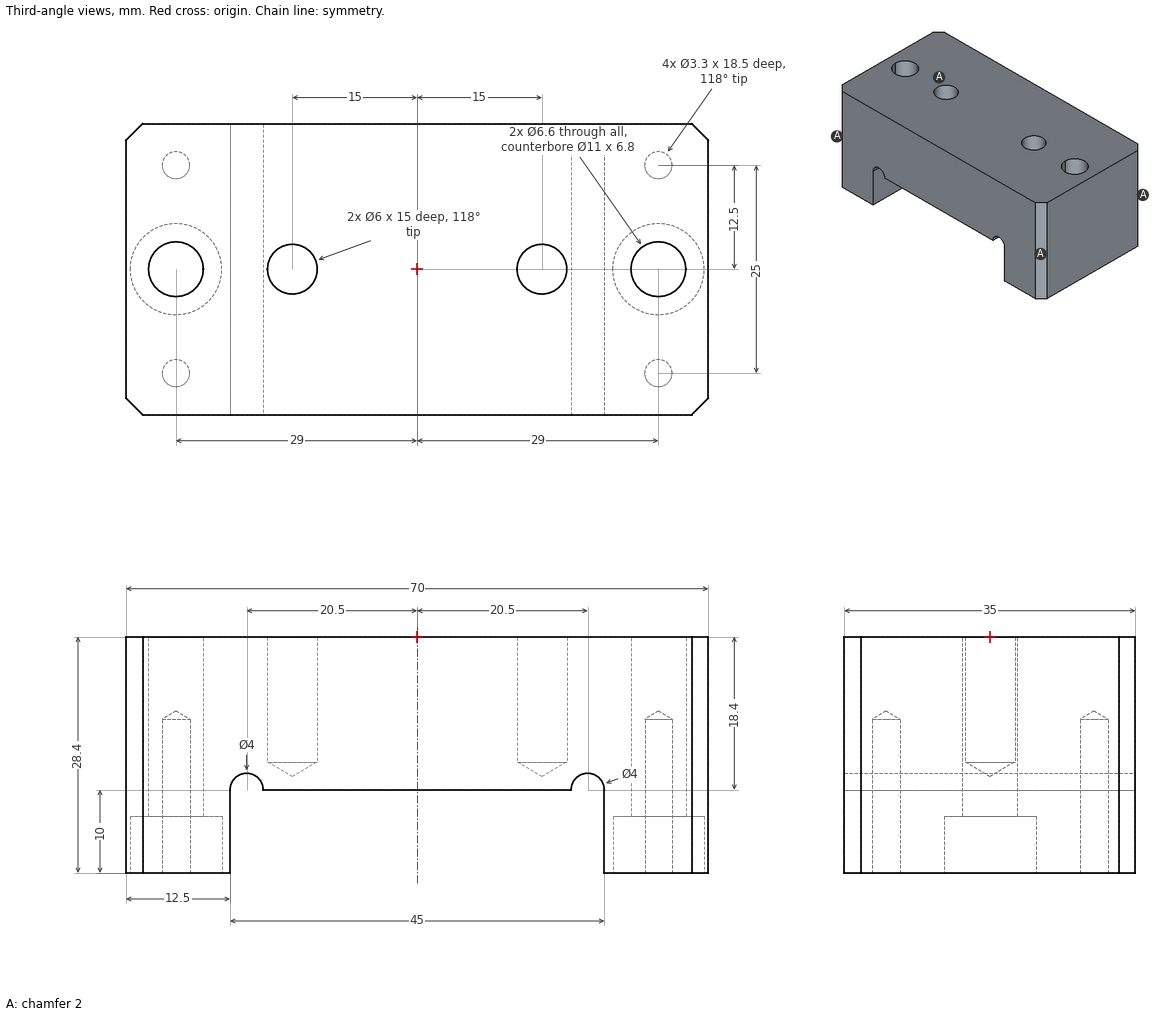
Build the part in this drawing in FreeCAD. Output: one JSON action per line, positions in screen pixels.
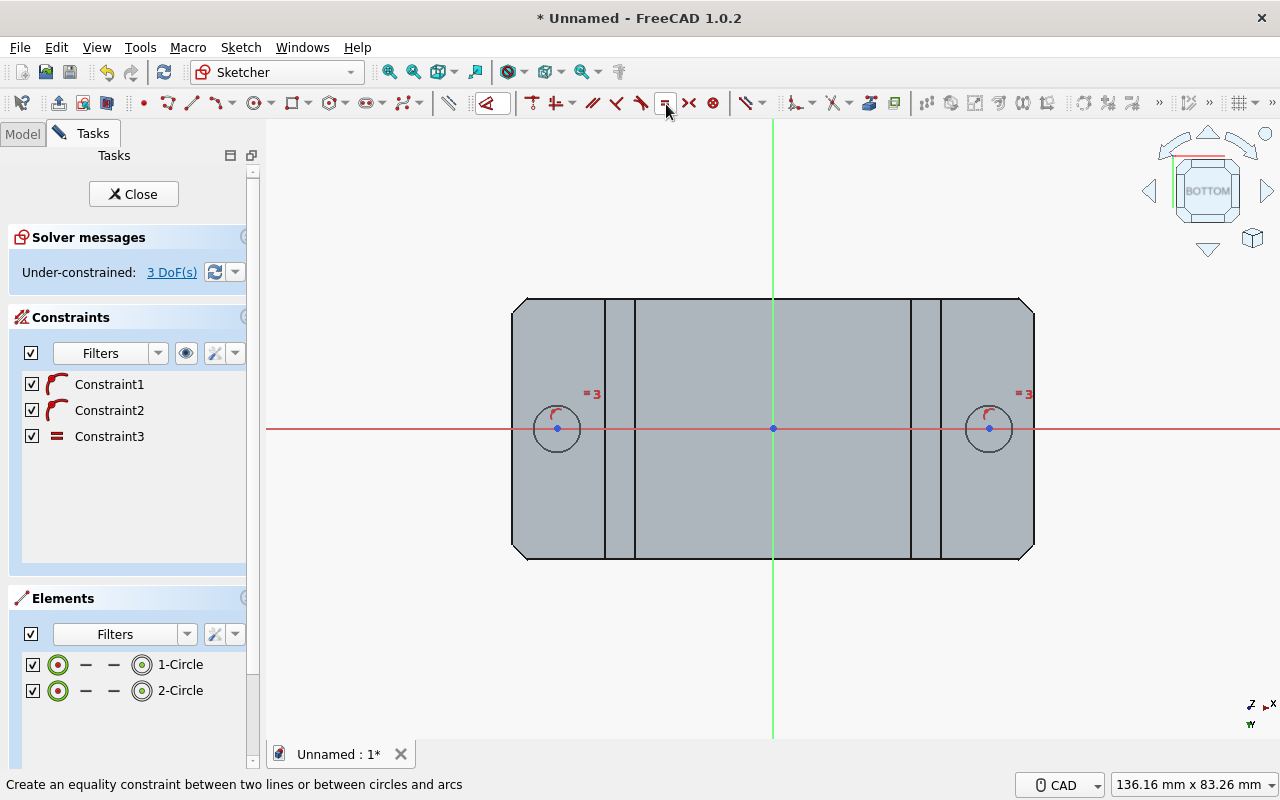
{"action": "left_click", "coordinate": [1005, 412]}
{"action": "left_click", "coordinate": [1027, 389]}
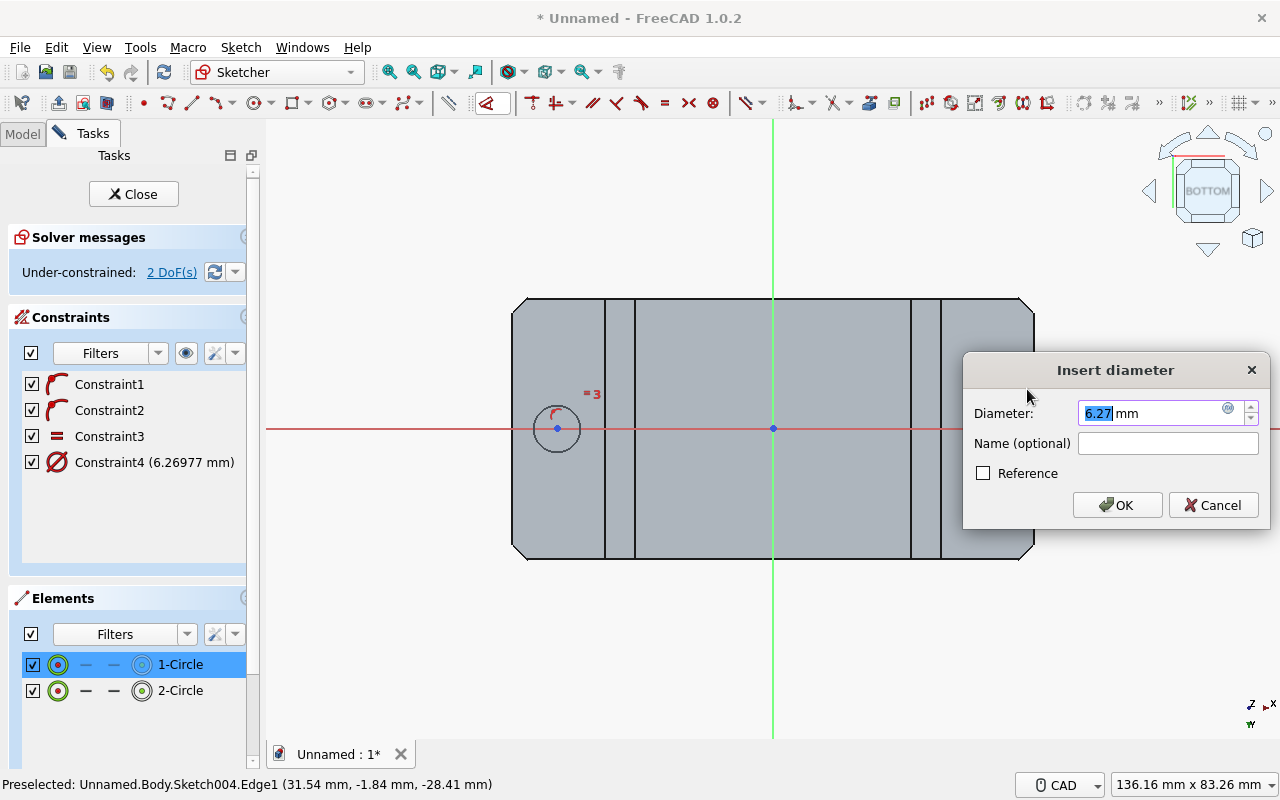
{"action": "type", "text": "6.6"}
{"action": "key", "text": "Return"}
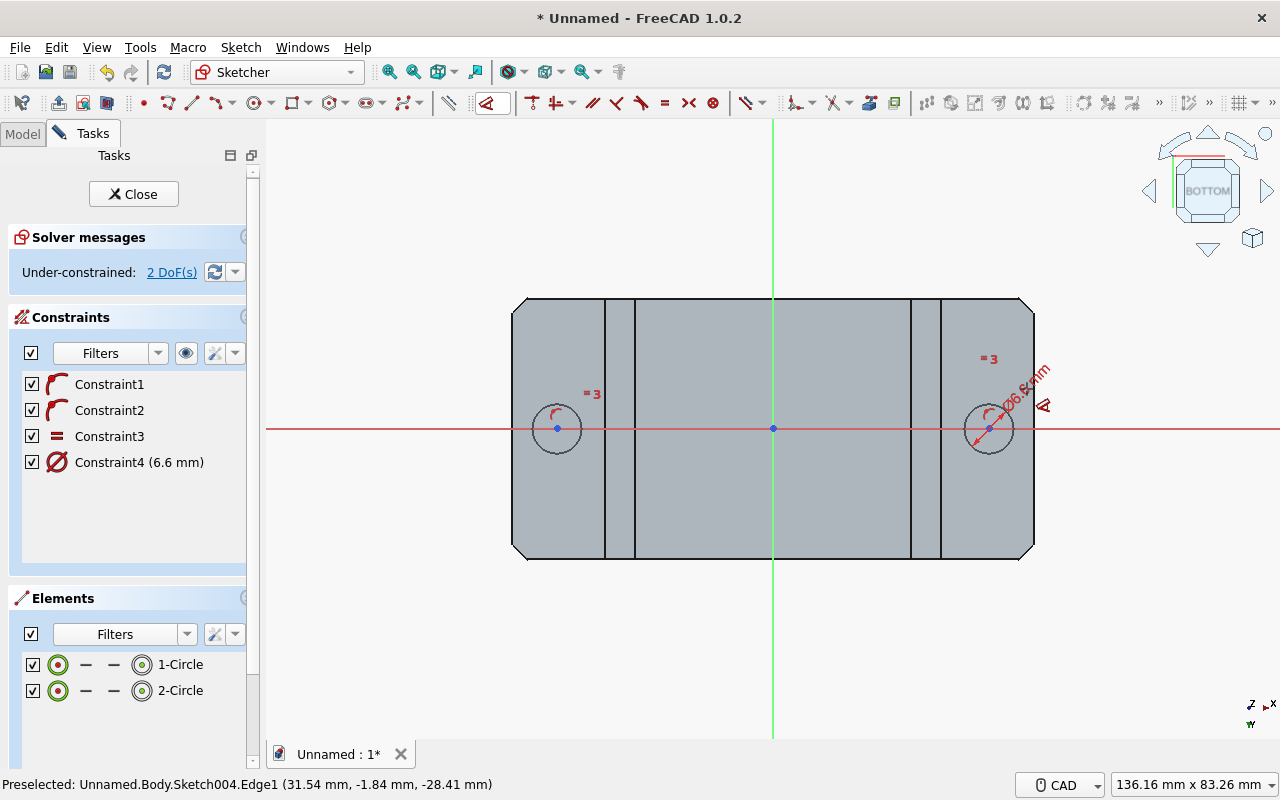
{"action": "left_click", "coordinate": [989, 429]}
{"action": "left_click", "coordinate": [881, 463]}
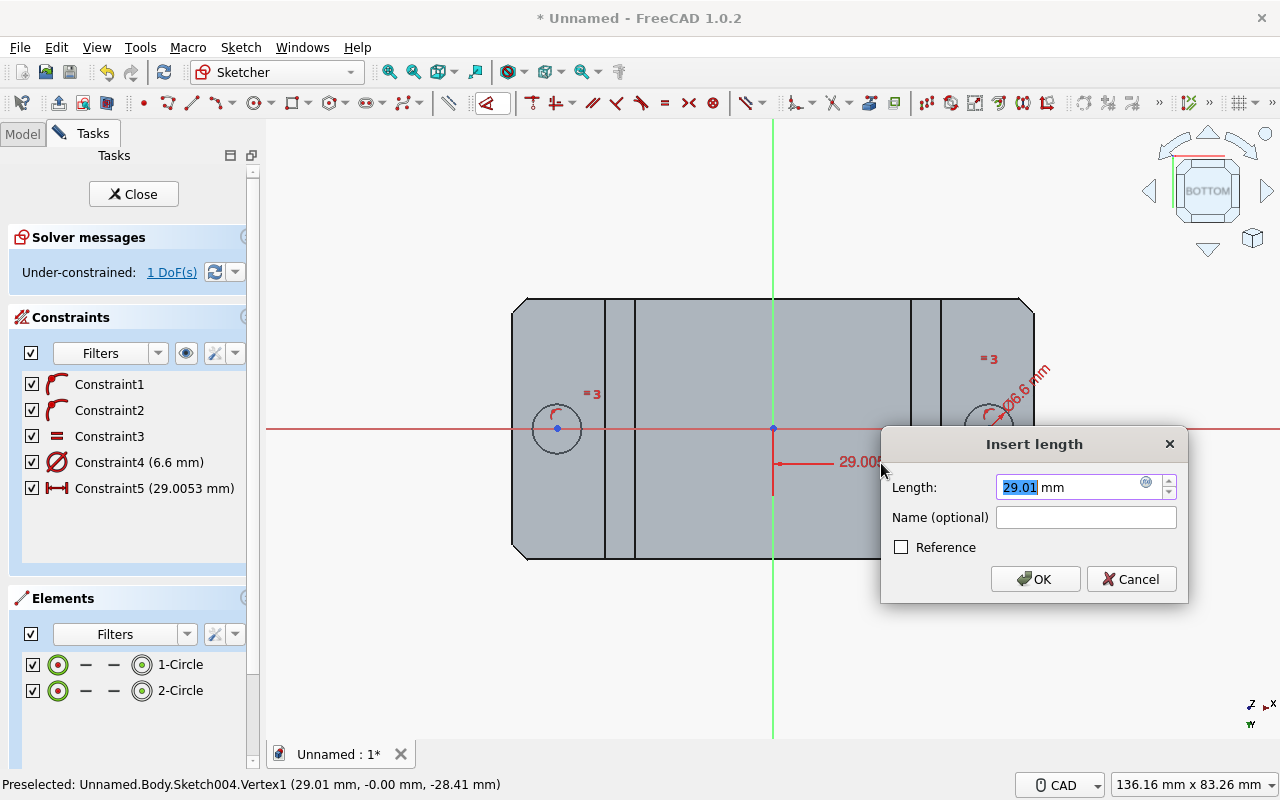
{"action": "type", "text": "29"}
{"action": "key", "text": "Return"}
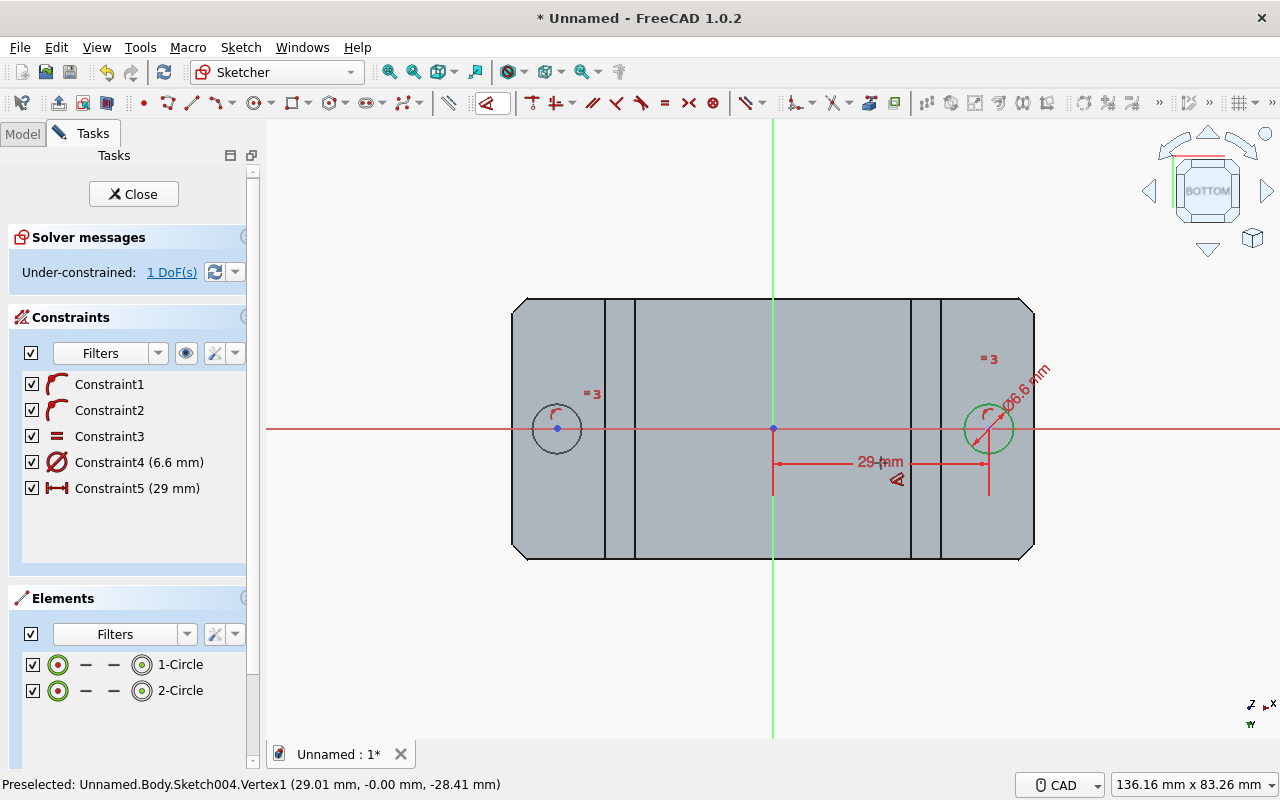
{"action": "left_click", "coordinate": [557, 429]}
{"action": "left_click", "coordinate": [665, 463]}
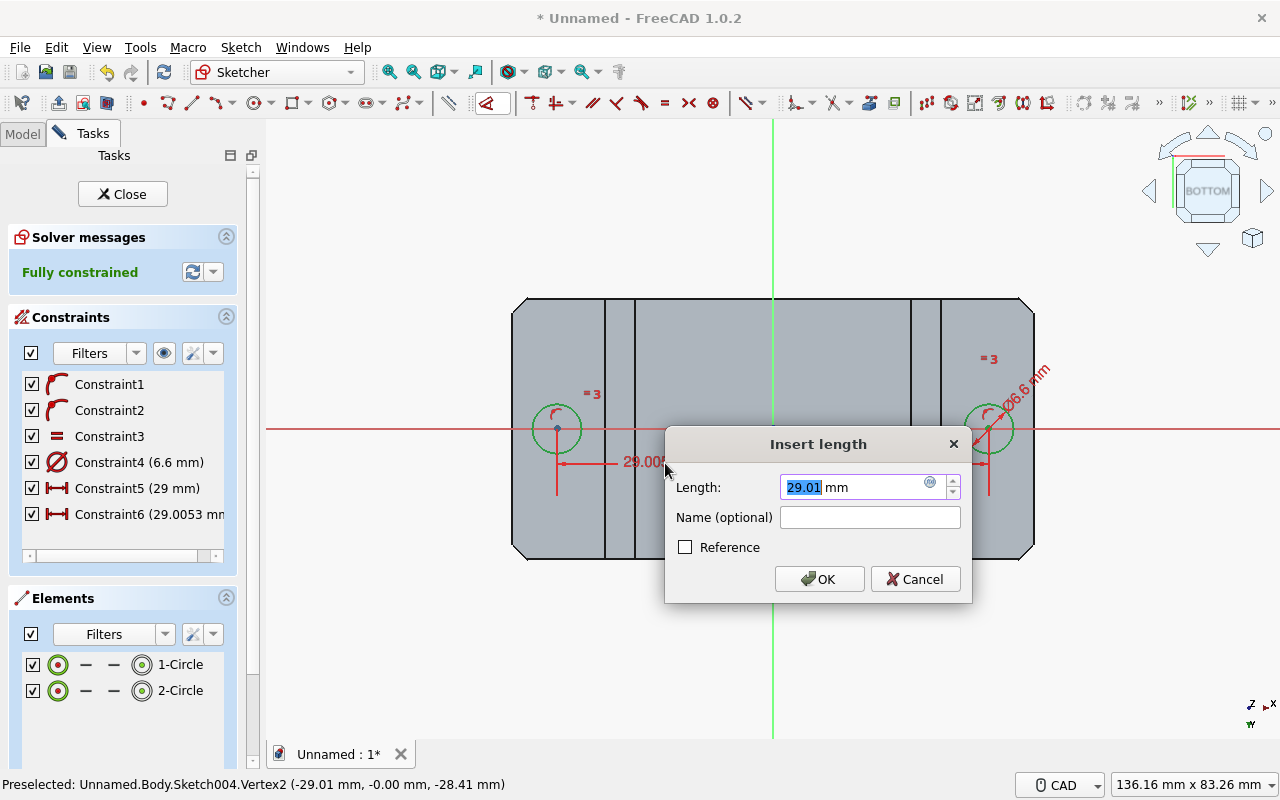
{"action": "type", "text": "29"}
{"action": "key", "text": "Return"}
{"action": "key", "text": "Escape"}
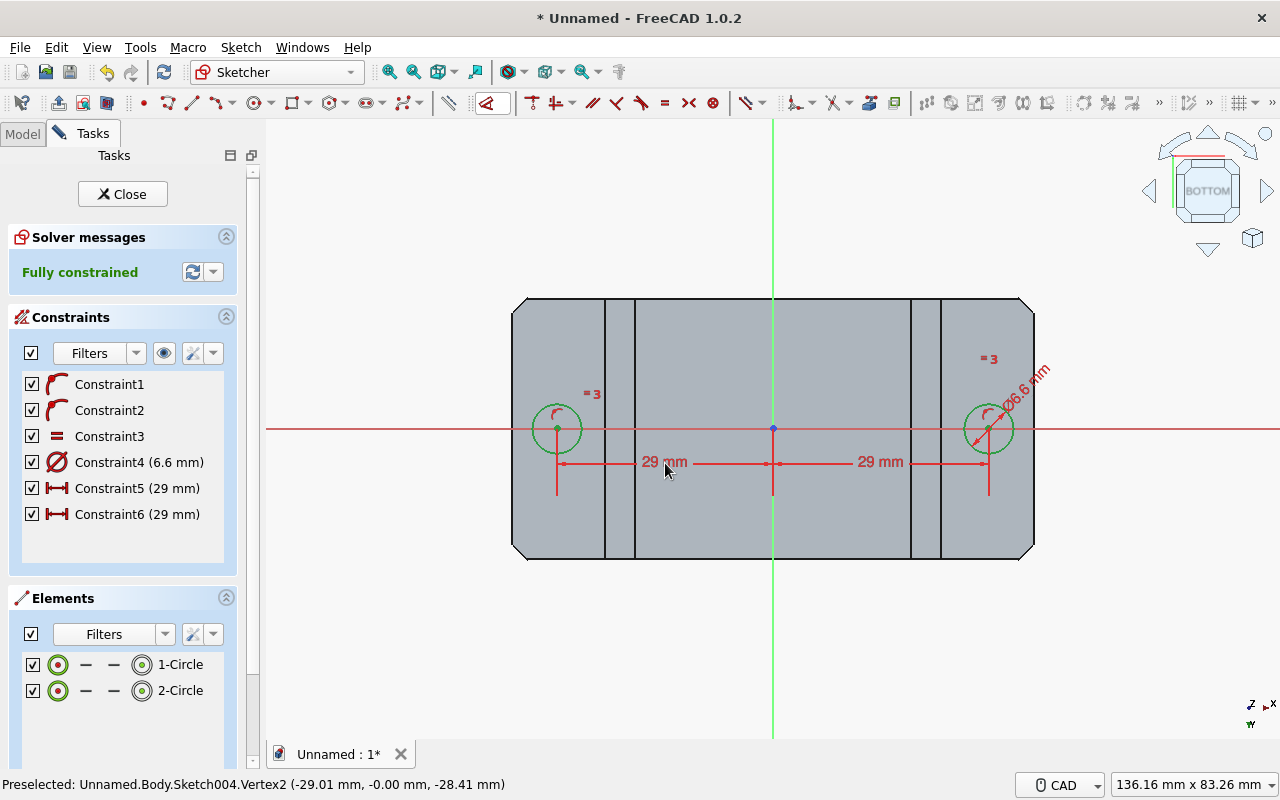
{"action": "left_click", "coordinate": [123, 194]}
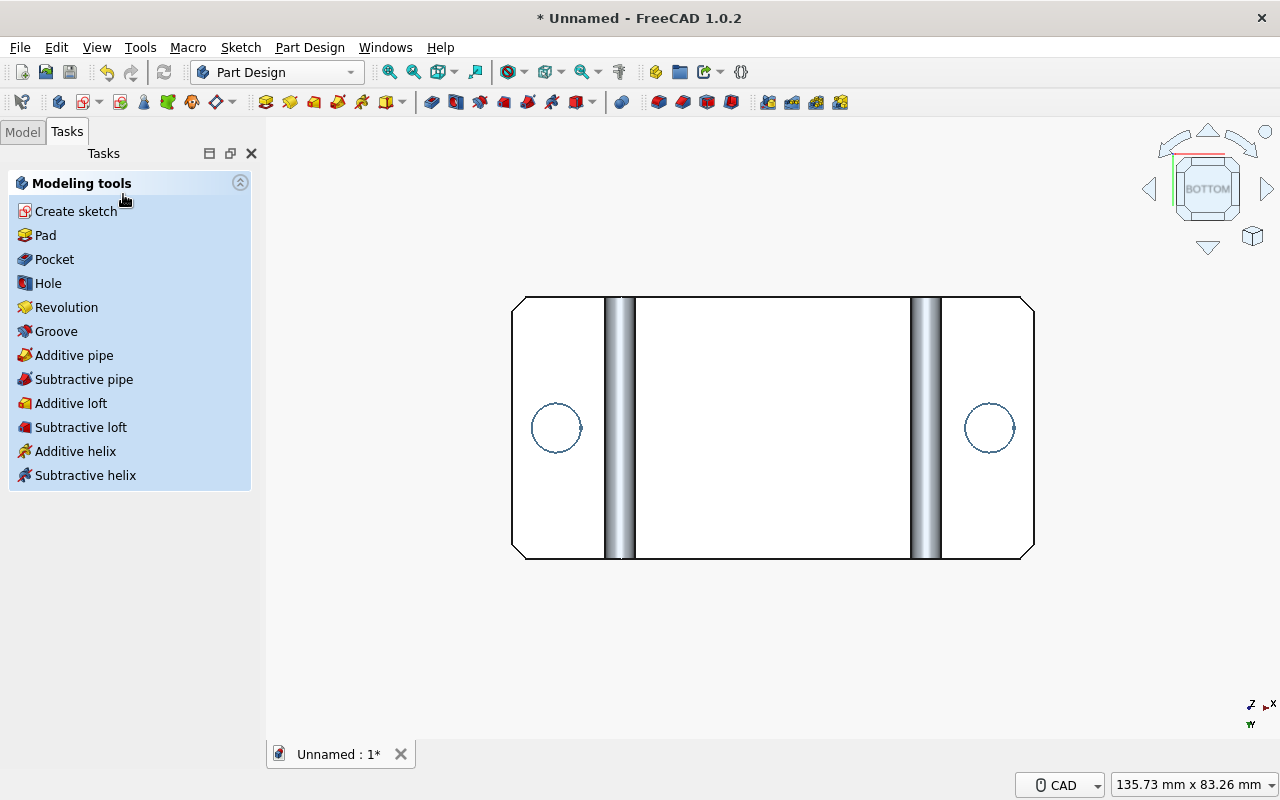
{"action": "left_click", "coordinate": [456, 102]}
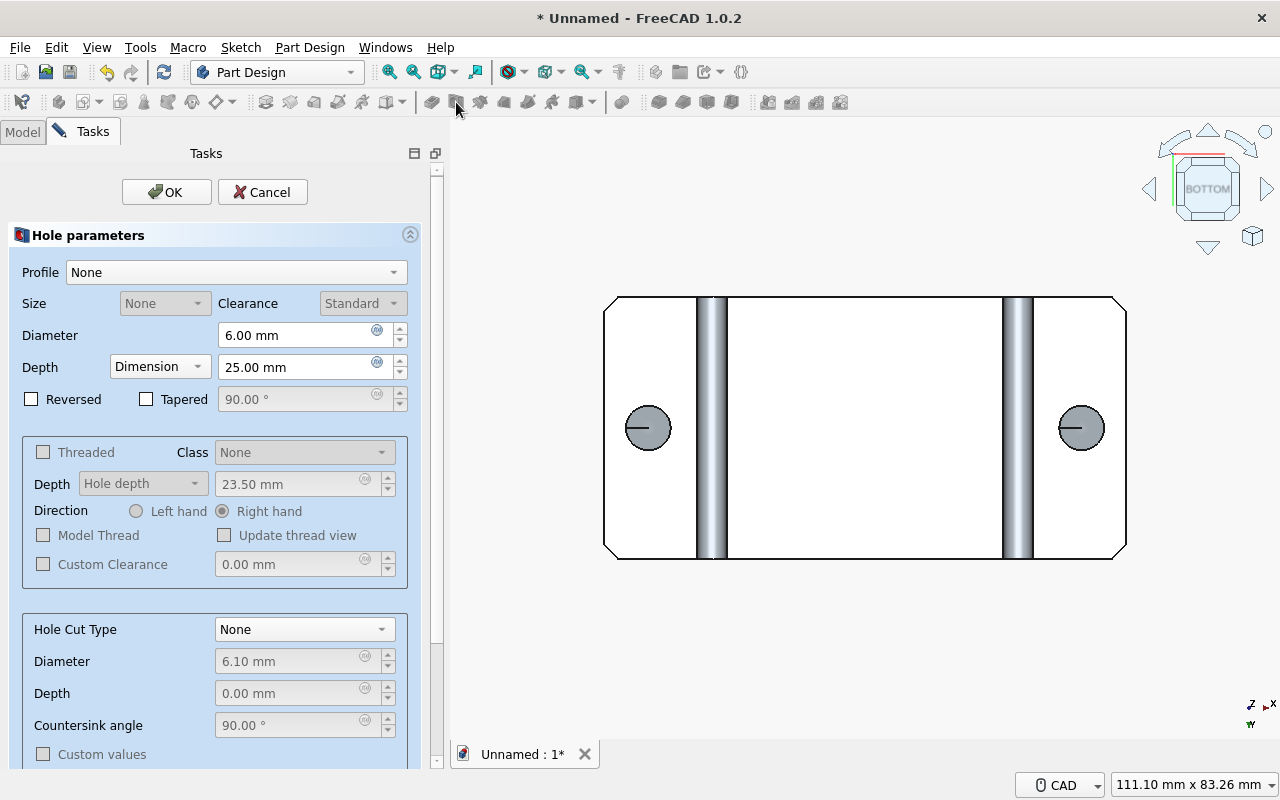
{"action": "triple_click", "coordinate": [305, 335]}